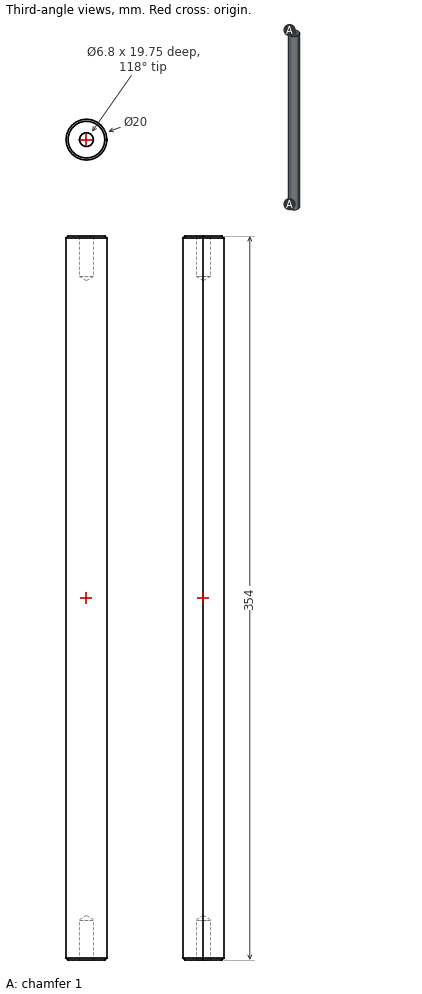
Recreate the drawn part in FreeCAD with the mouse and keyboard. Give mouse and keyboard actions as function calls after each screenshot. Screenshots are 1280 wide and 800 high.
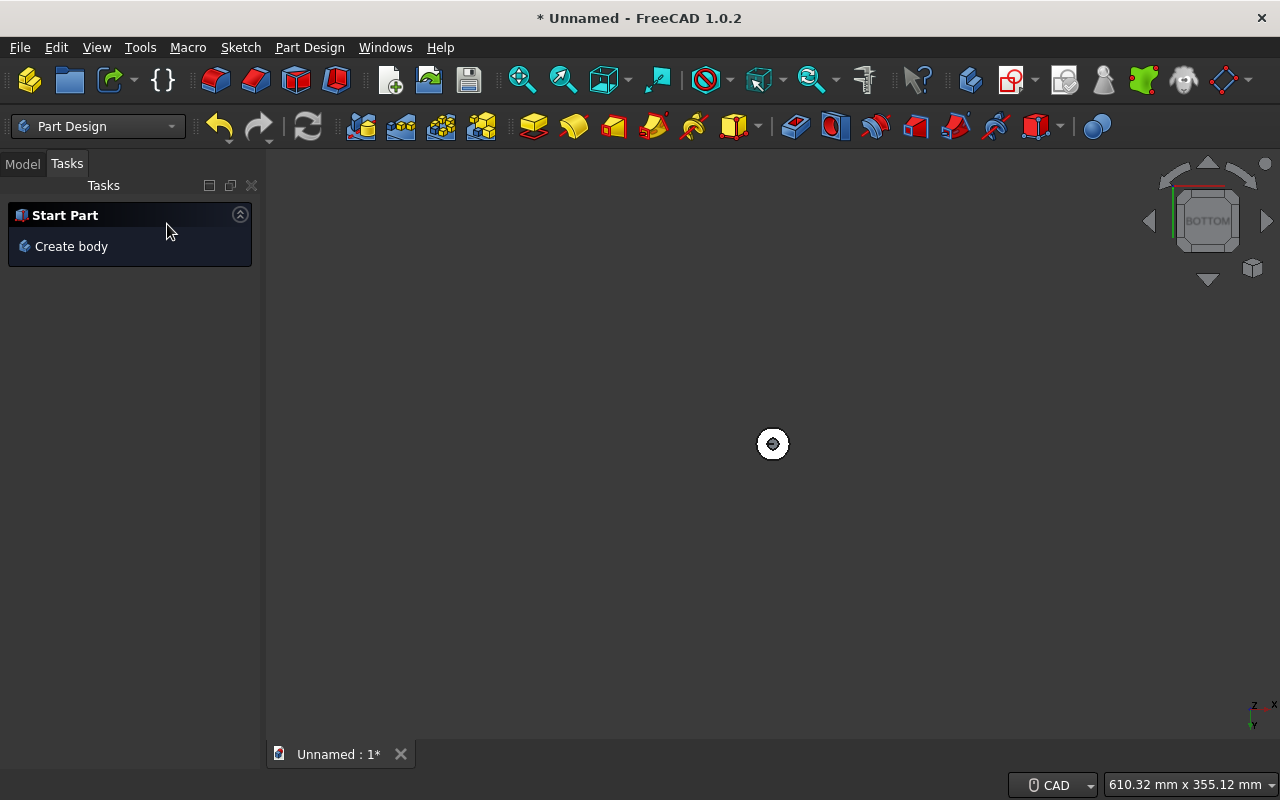
key(v)
key(f)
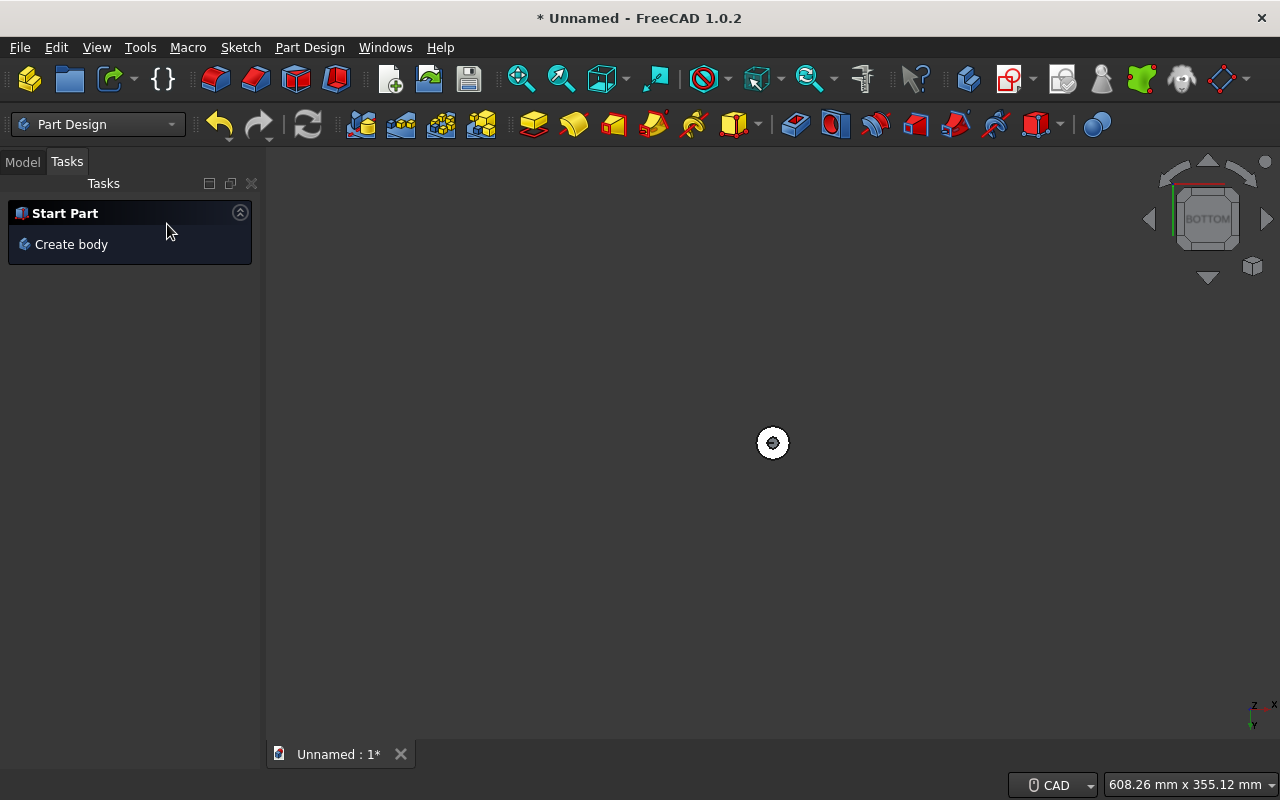
key(0)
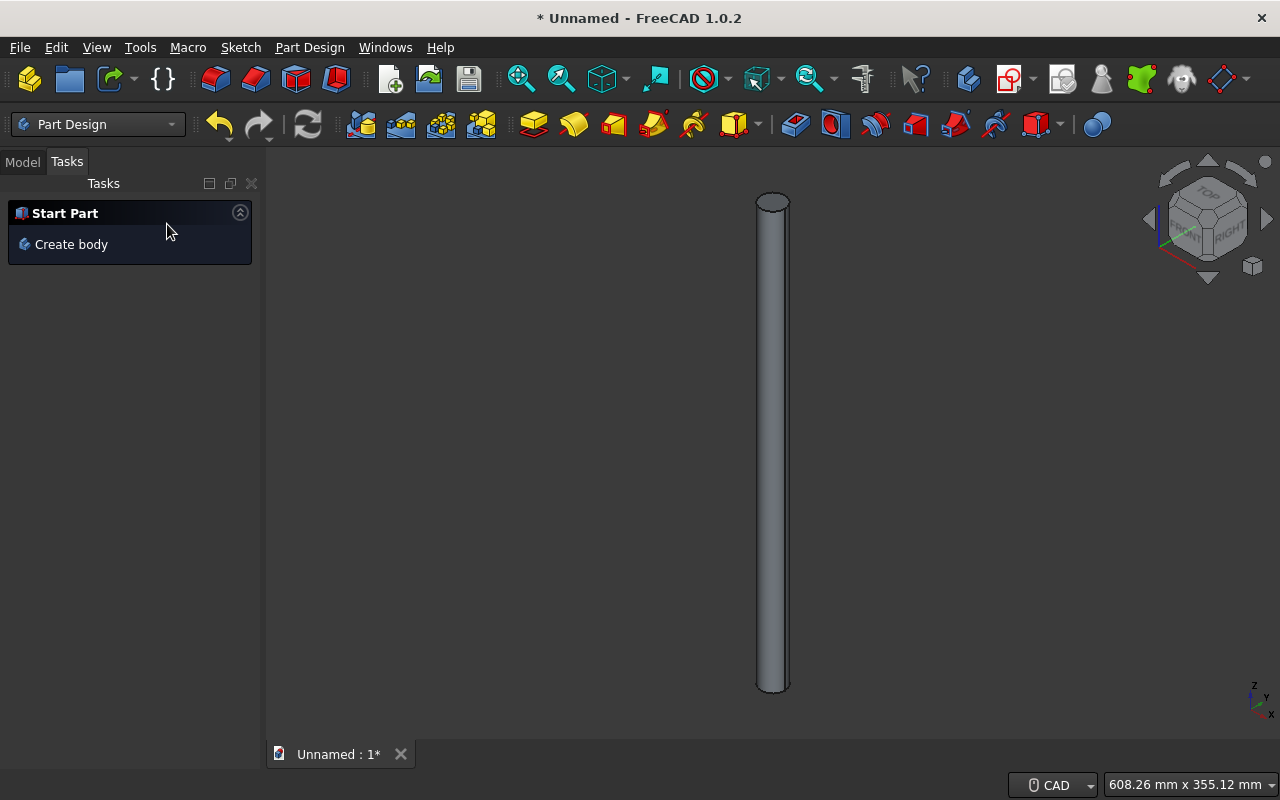
click(773, 201)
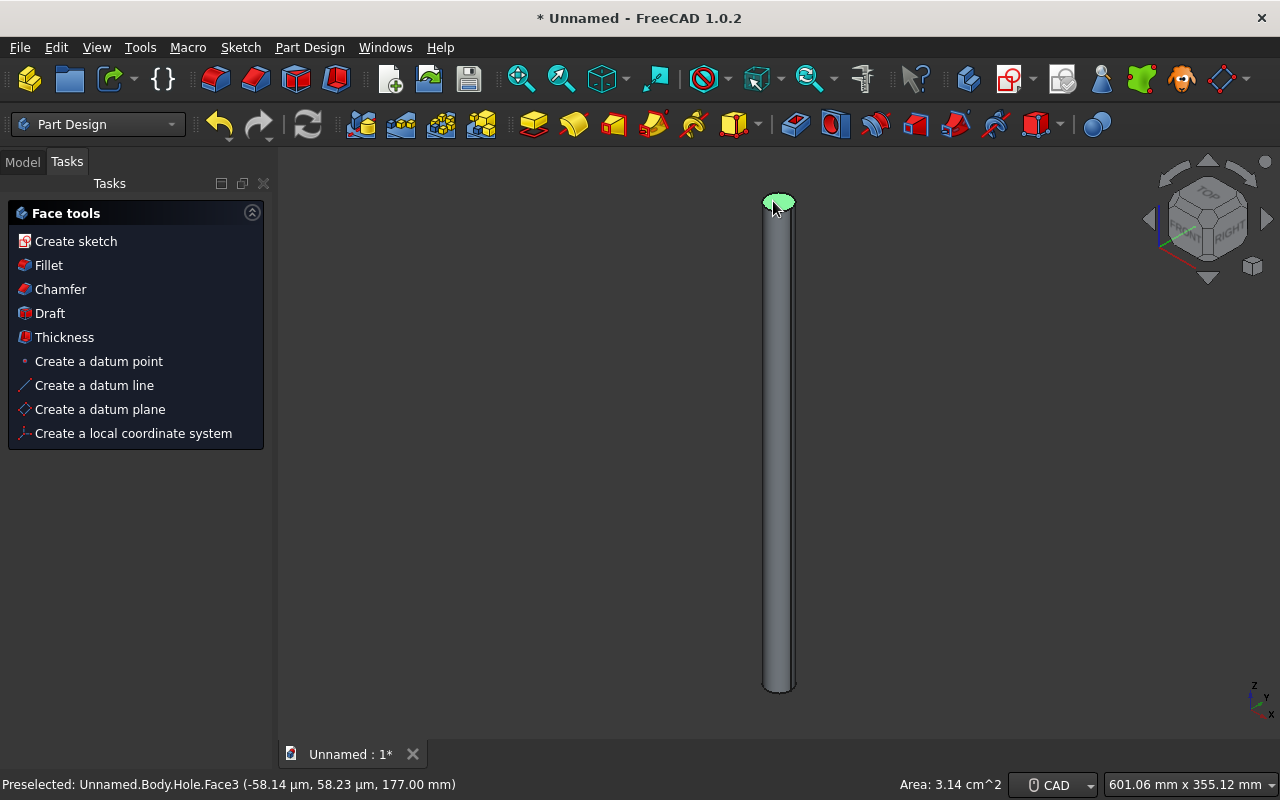
click(1010, 80)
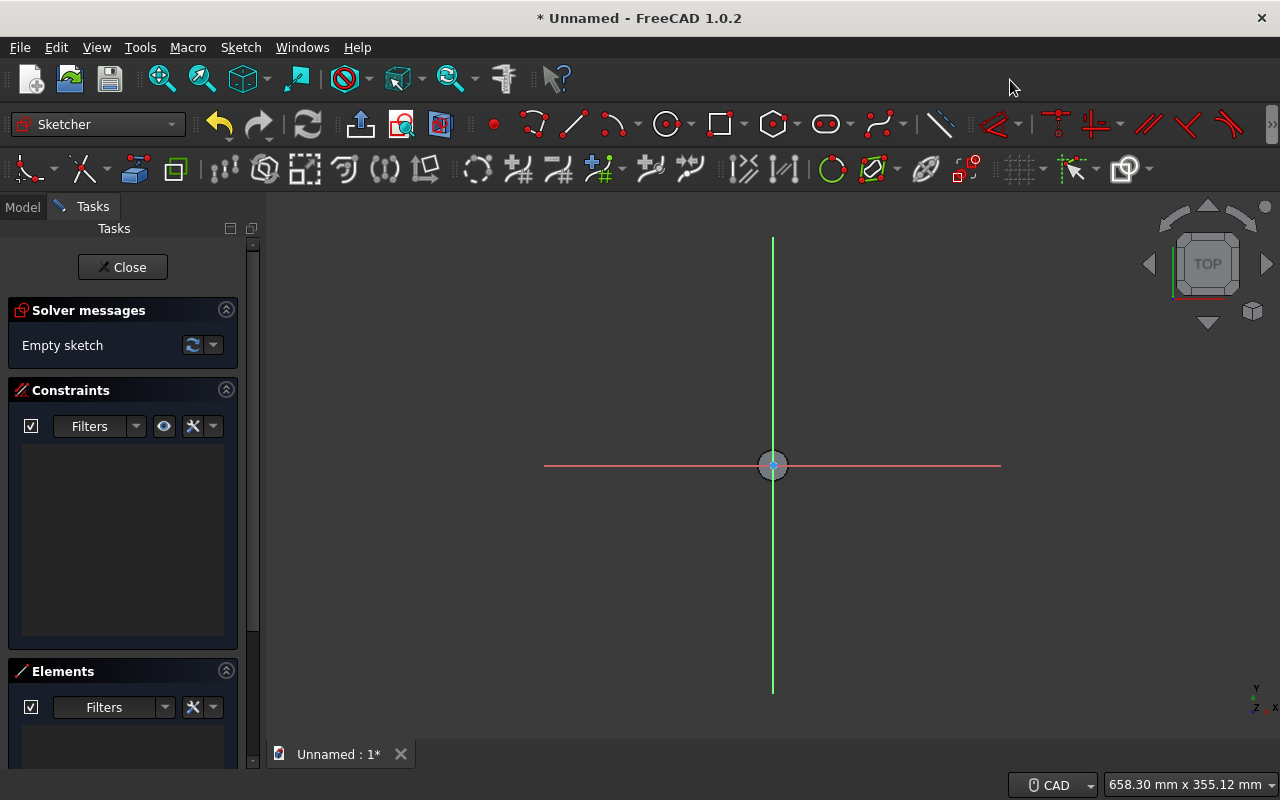
scroll(777, 466, up, 15)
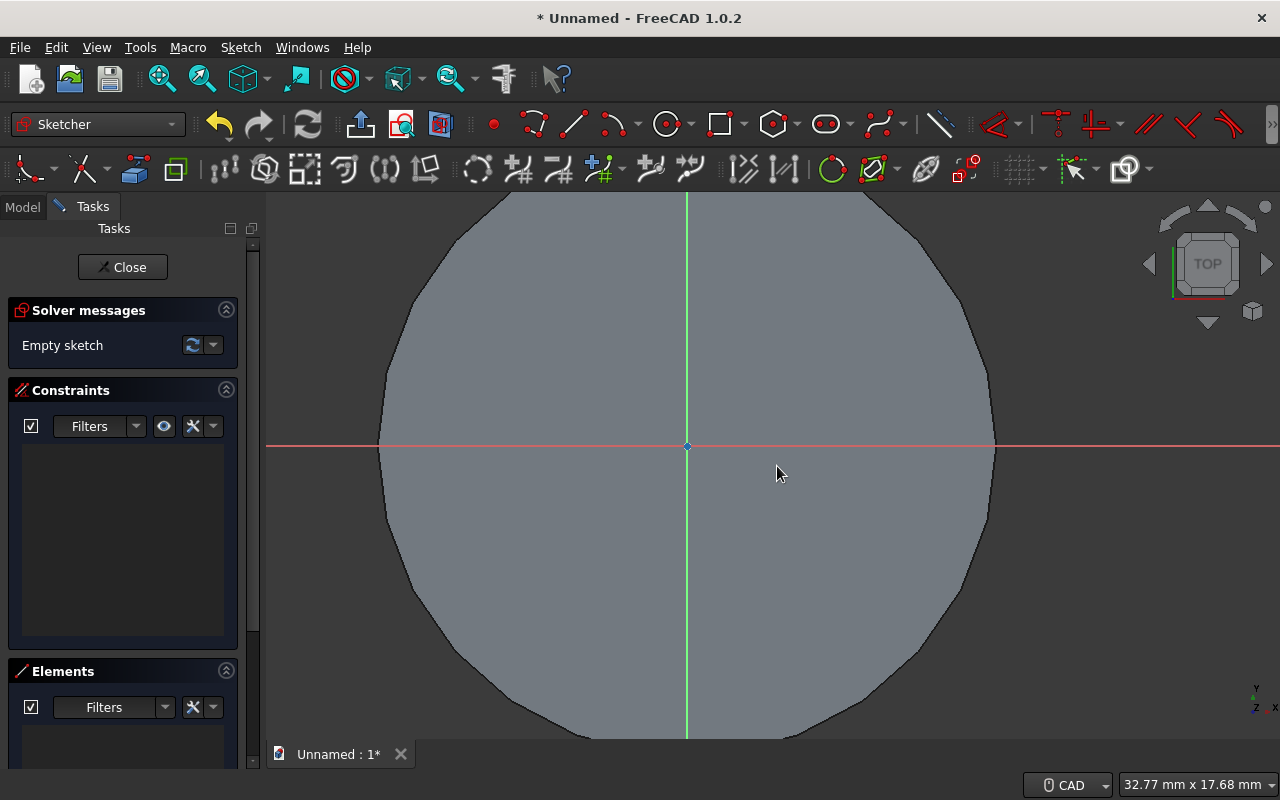
scroll(652, 408, up, 2)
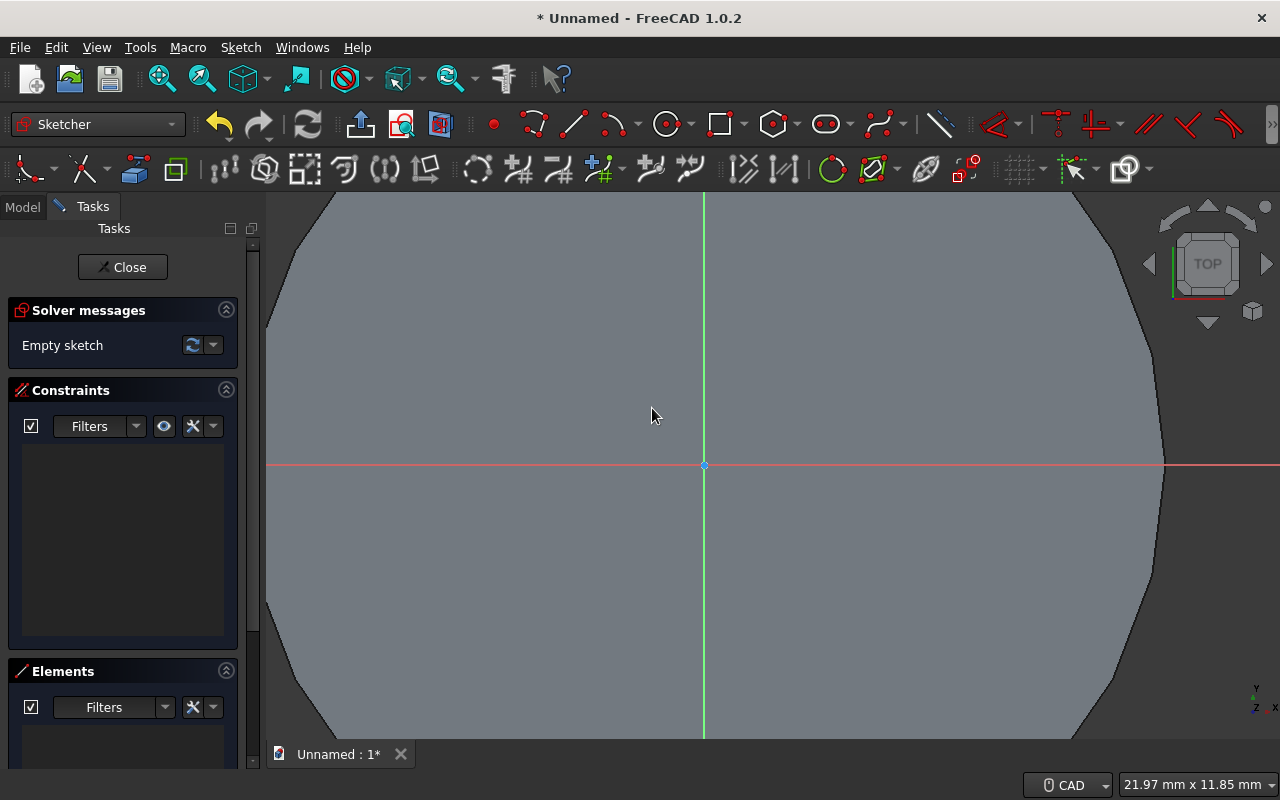
key(g)
key(c)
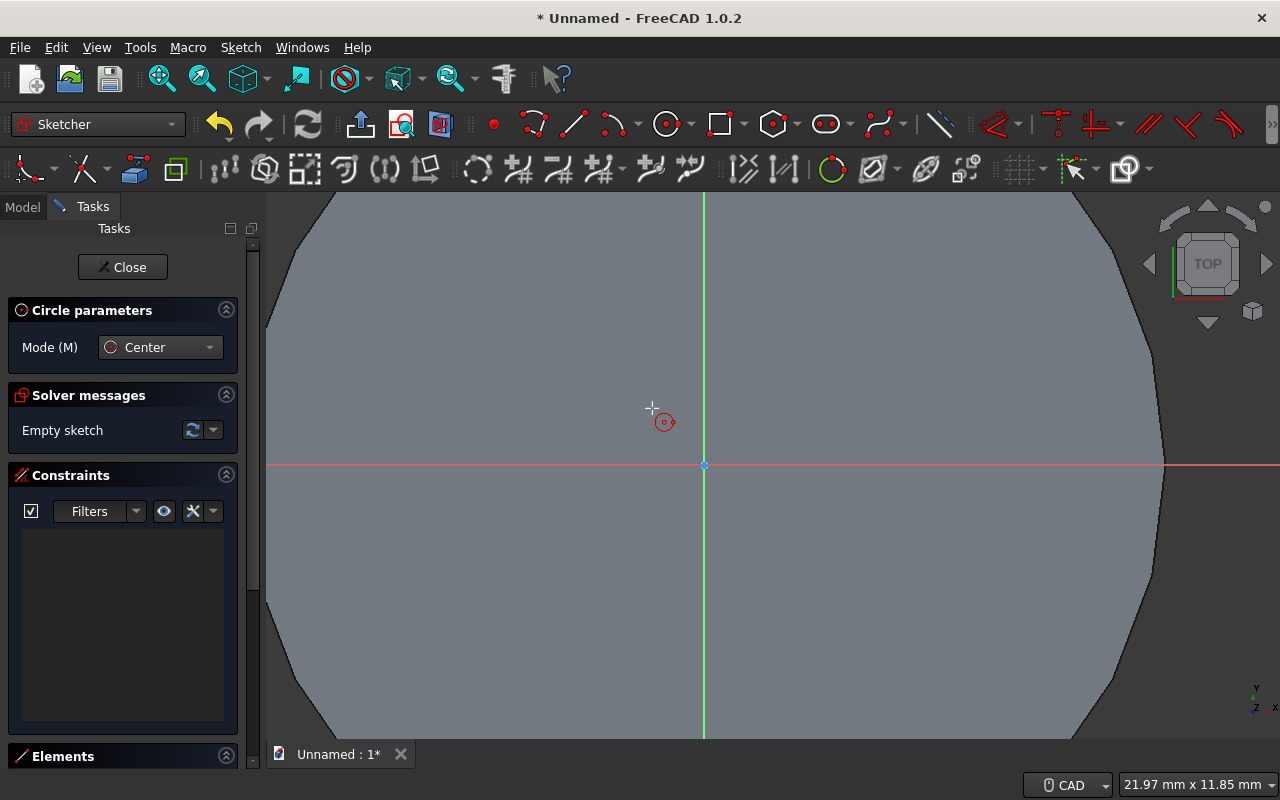
click(704, 465)
move(815, 354)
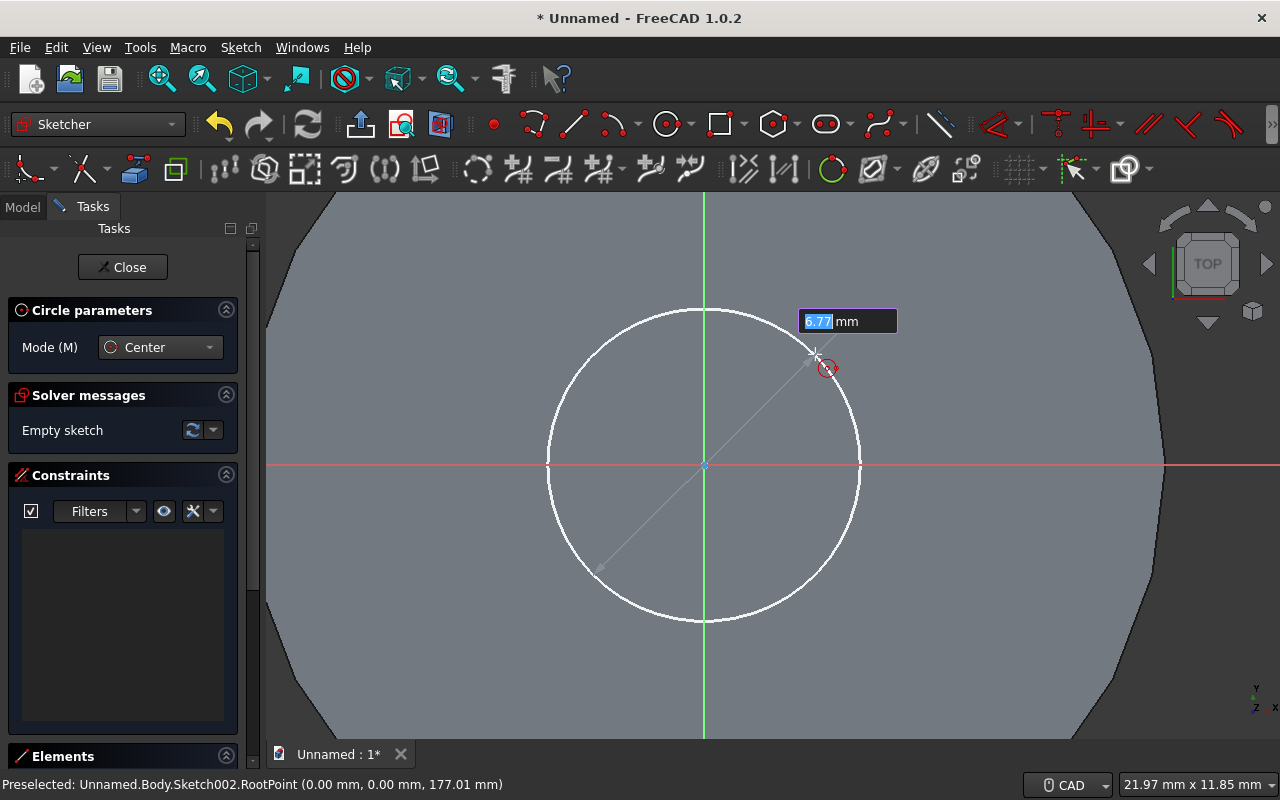
text(6.8)
key(Return)
key(Escape)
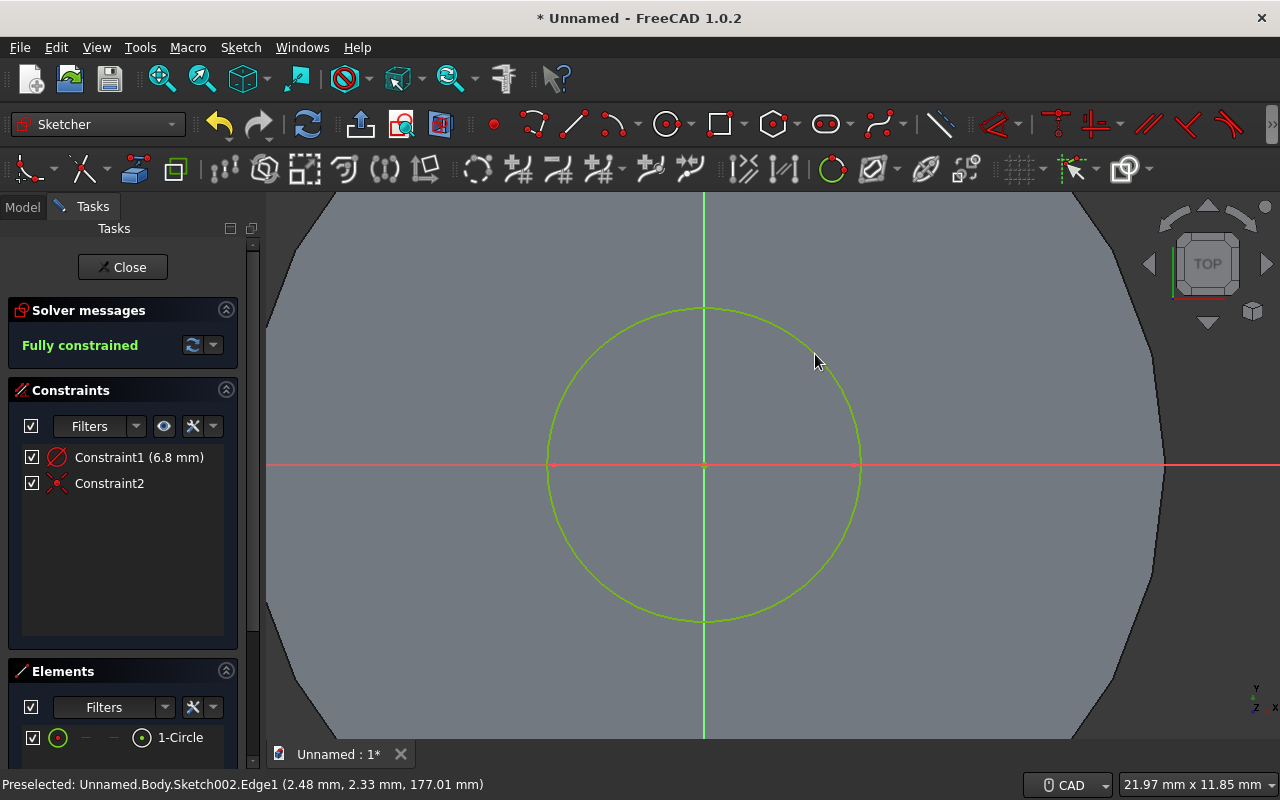
click(123, 267)